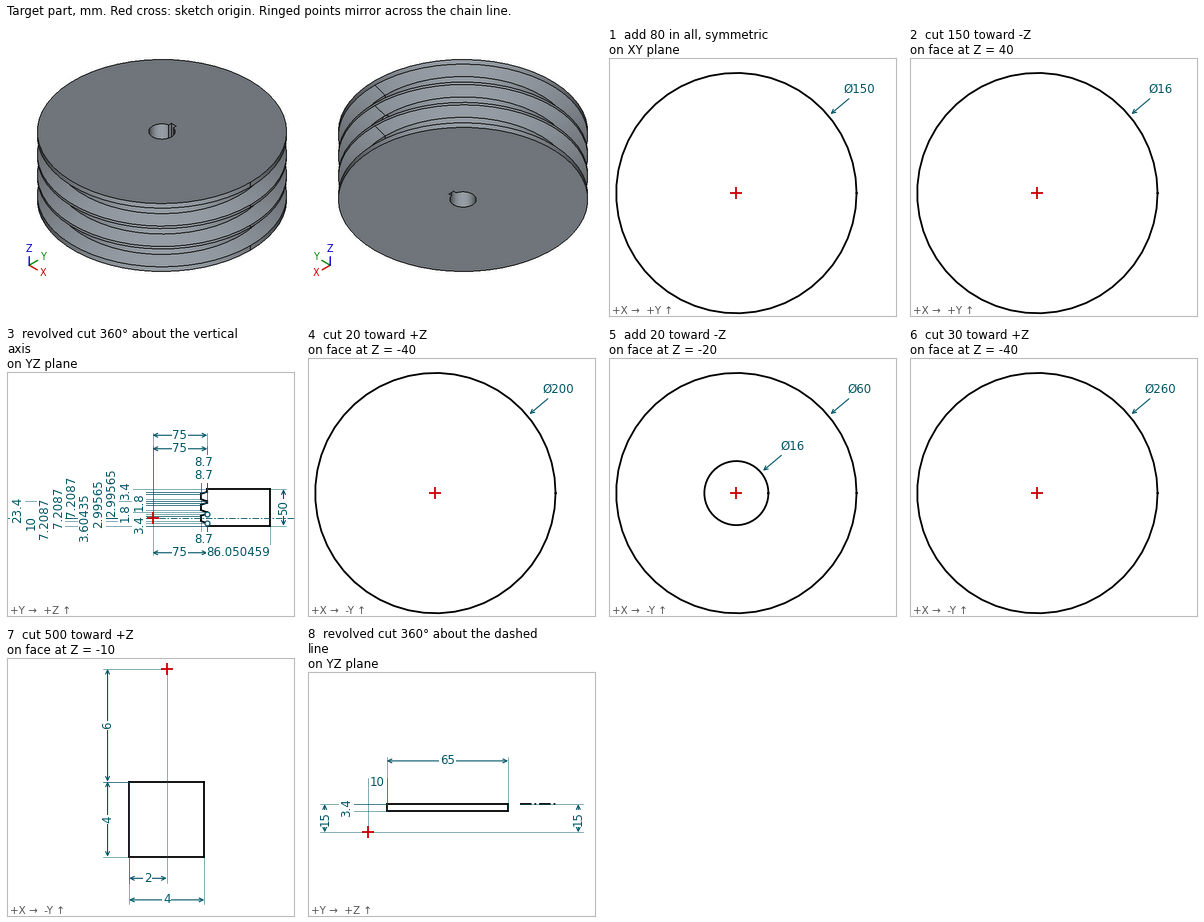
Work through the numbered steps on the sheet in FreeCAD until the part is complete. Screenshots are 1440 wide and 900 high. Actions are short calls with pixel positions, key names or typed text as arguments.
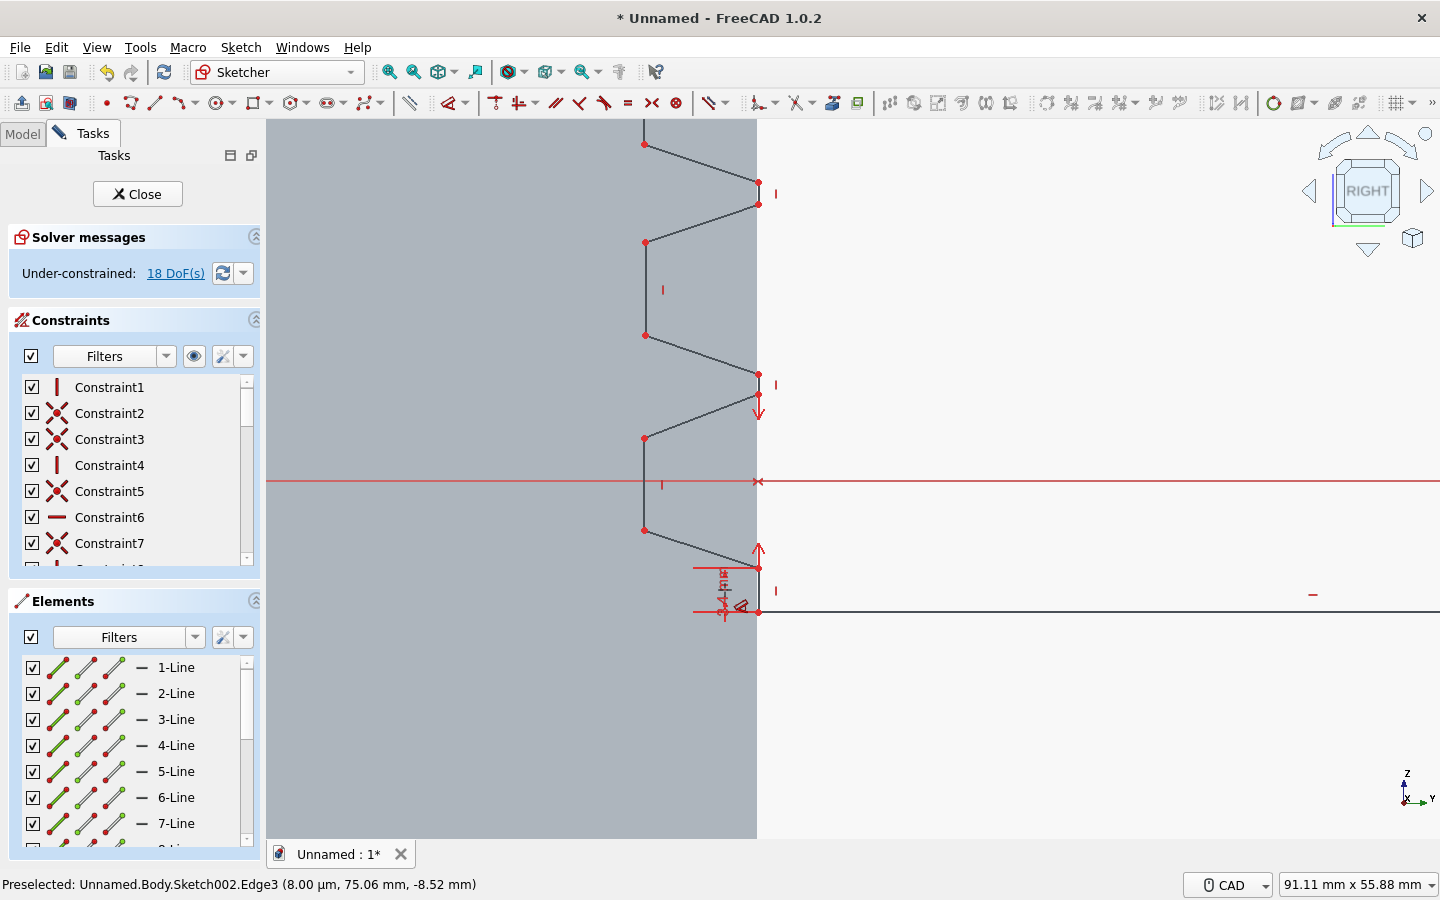
scroll(759, 590, down, 5)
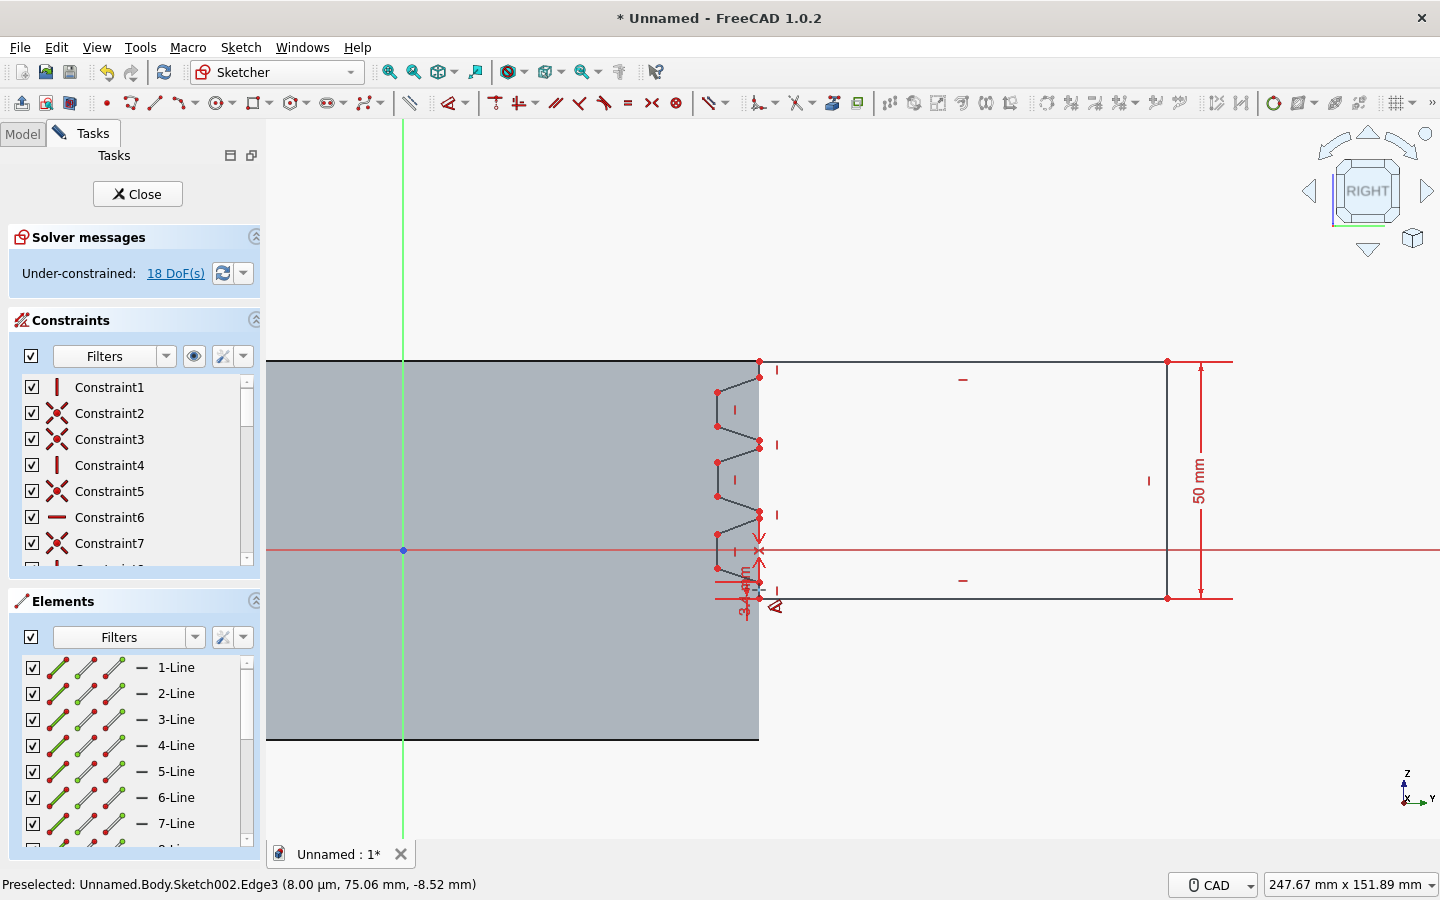
scroll(759, 366, up, 6)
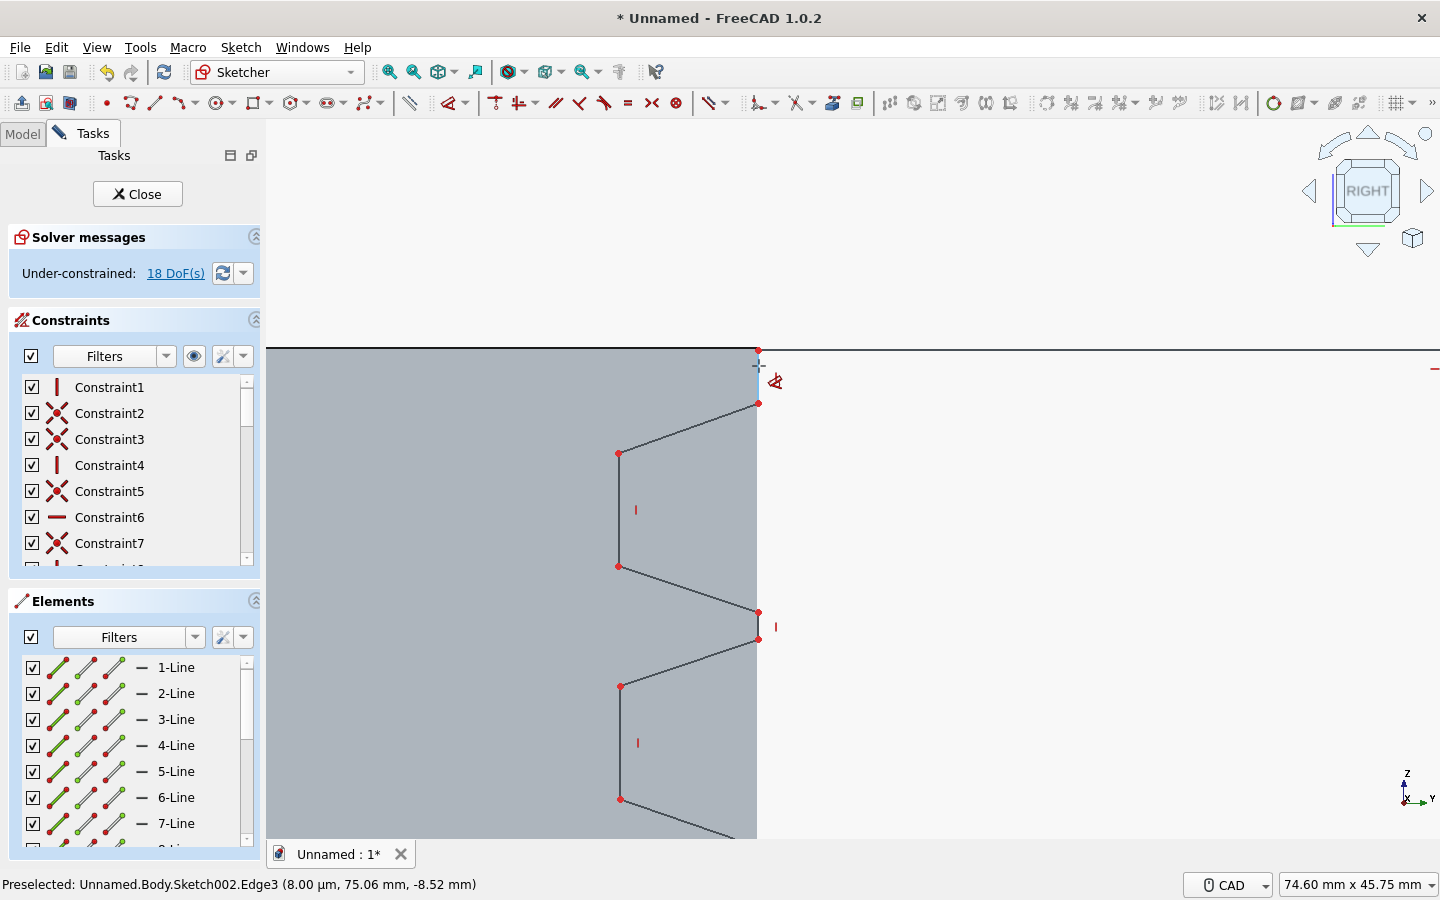
click(758, 366)
click(724, 377)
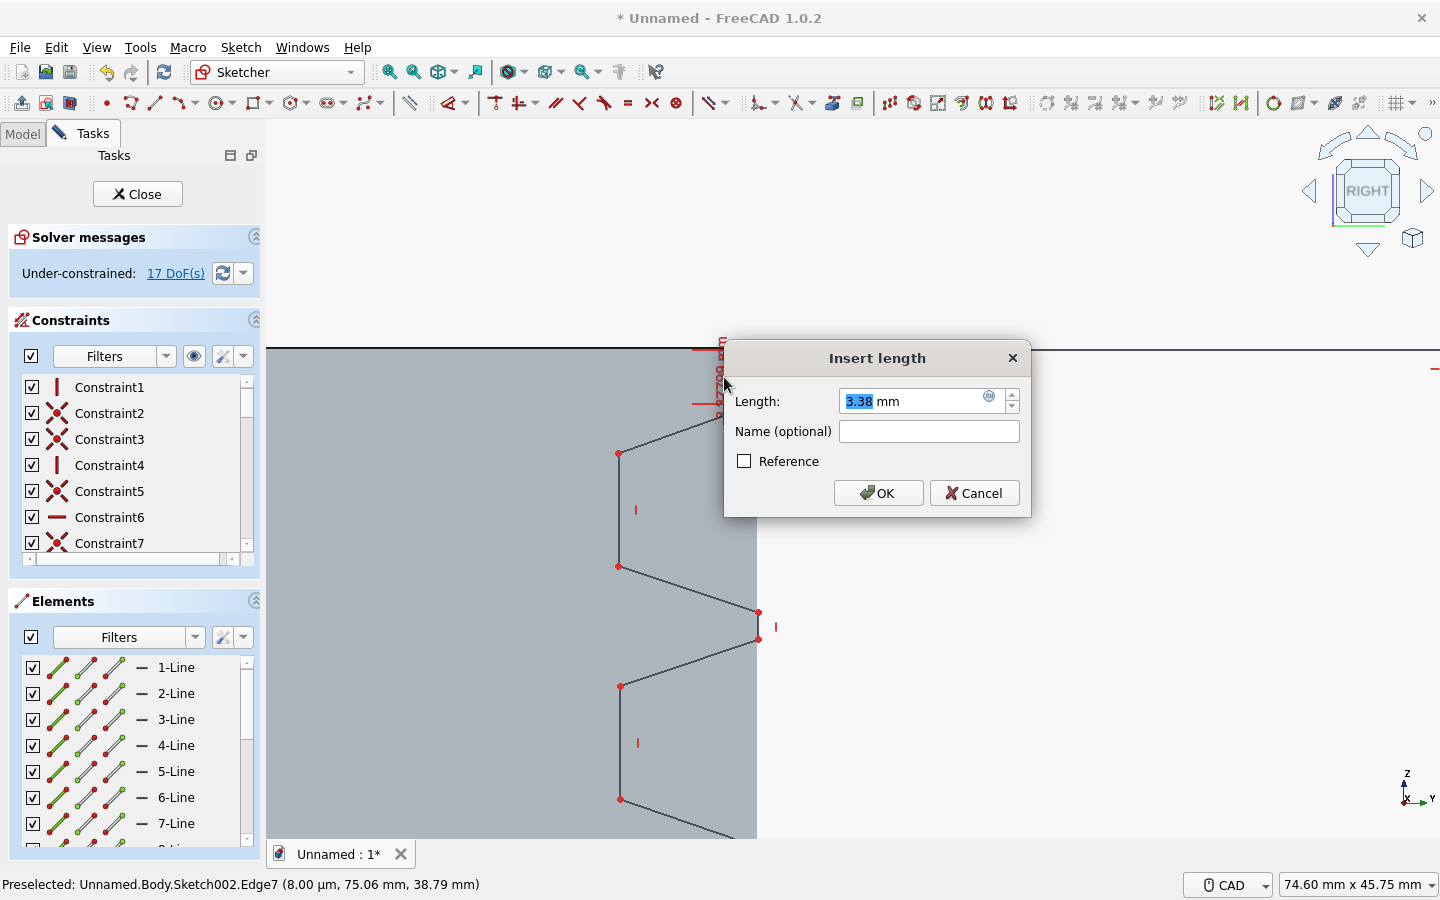
text(3.4)
key(Return)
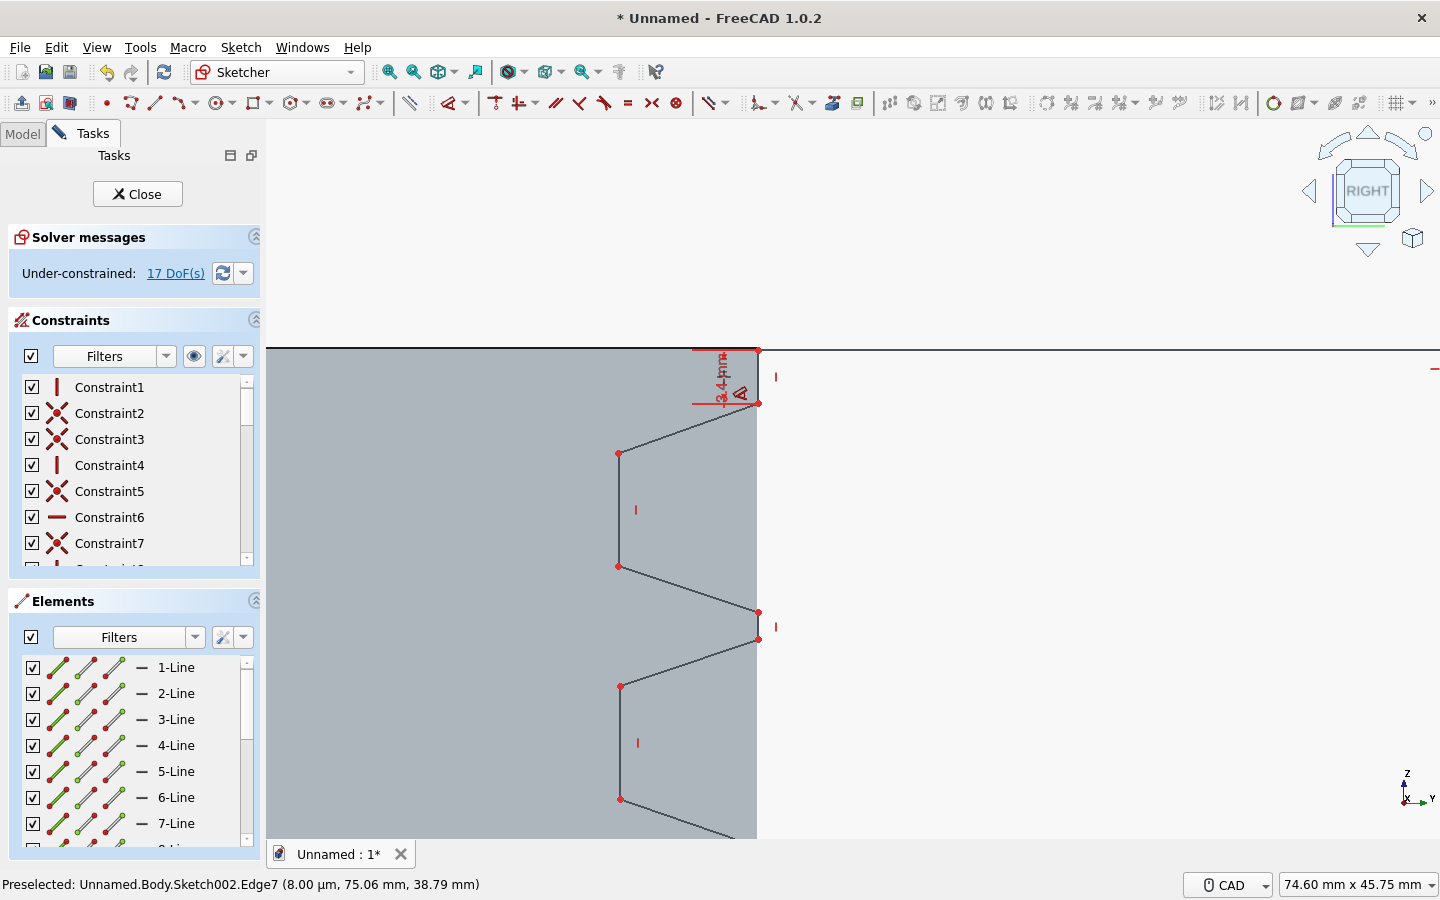
scroll(758, 624, up, 2)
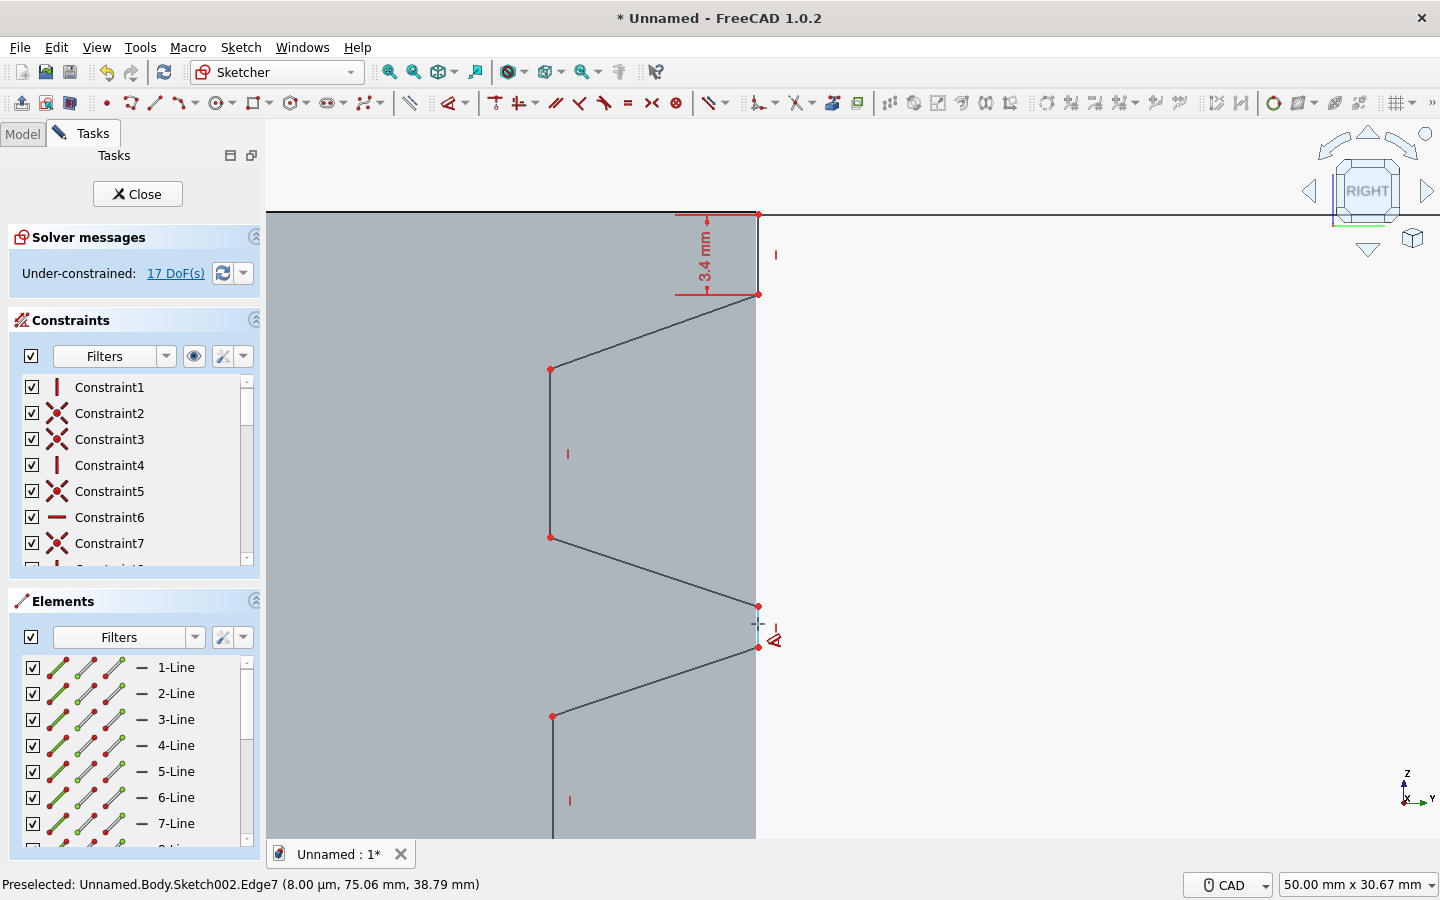
click(758, 623)
click(724, 627)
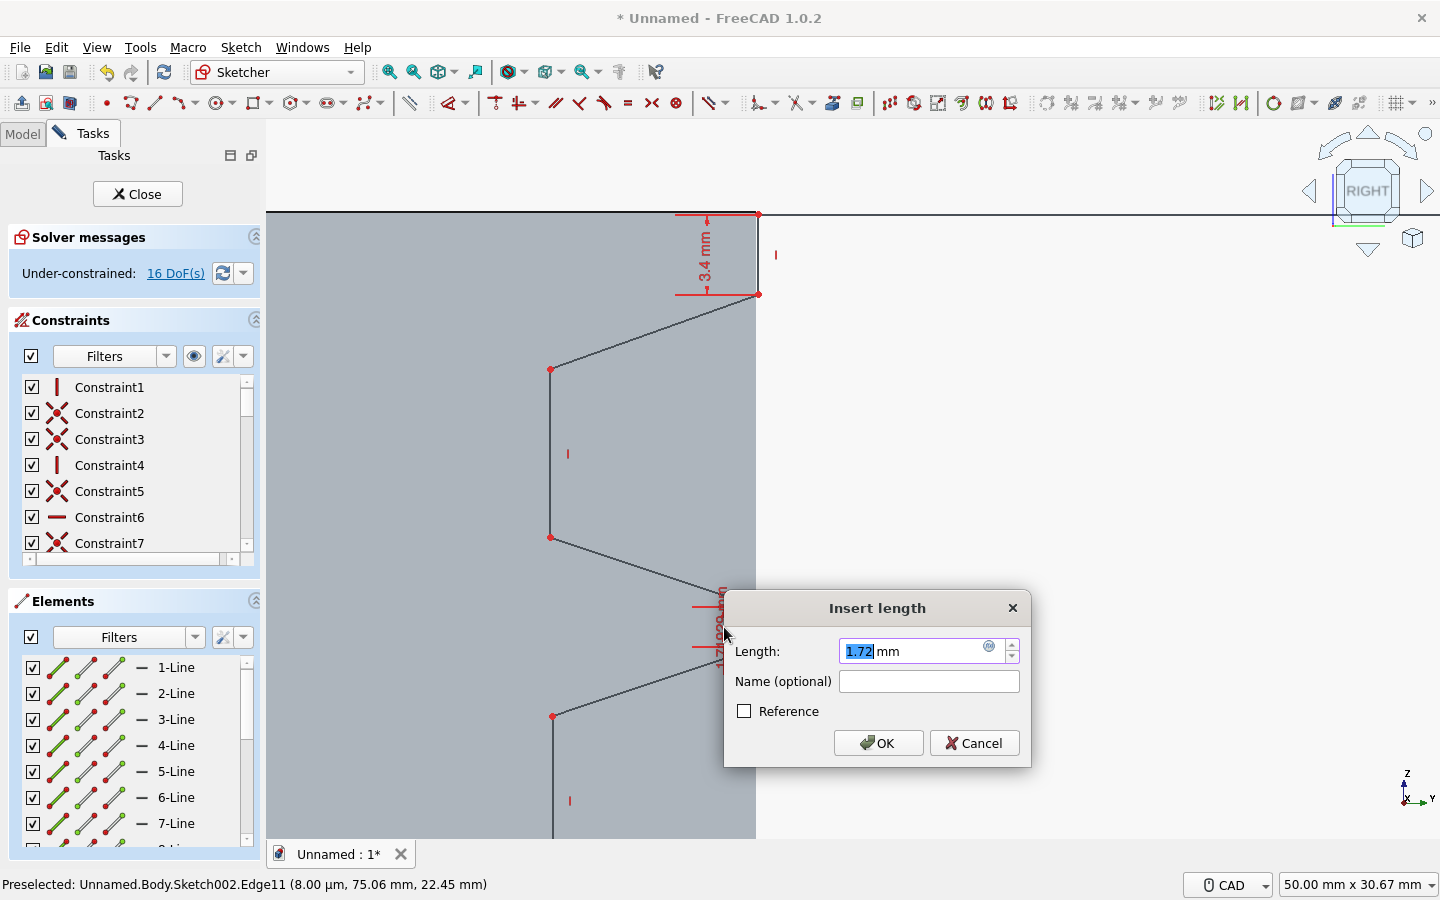
text(1.8)
key(Return)